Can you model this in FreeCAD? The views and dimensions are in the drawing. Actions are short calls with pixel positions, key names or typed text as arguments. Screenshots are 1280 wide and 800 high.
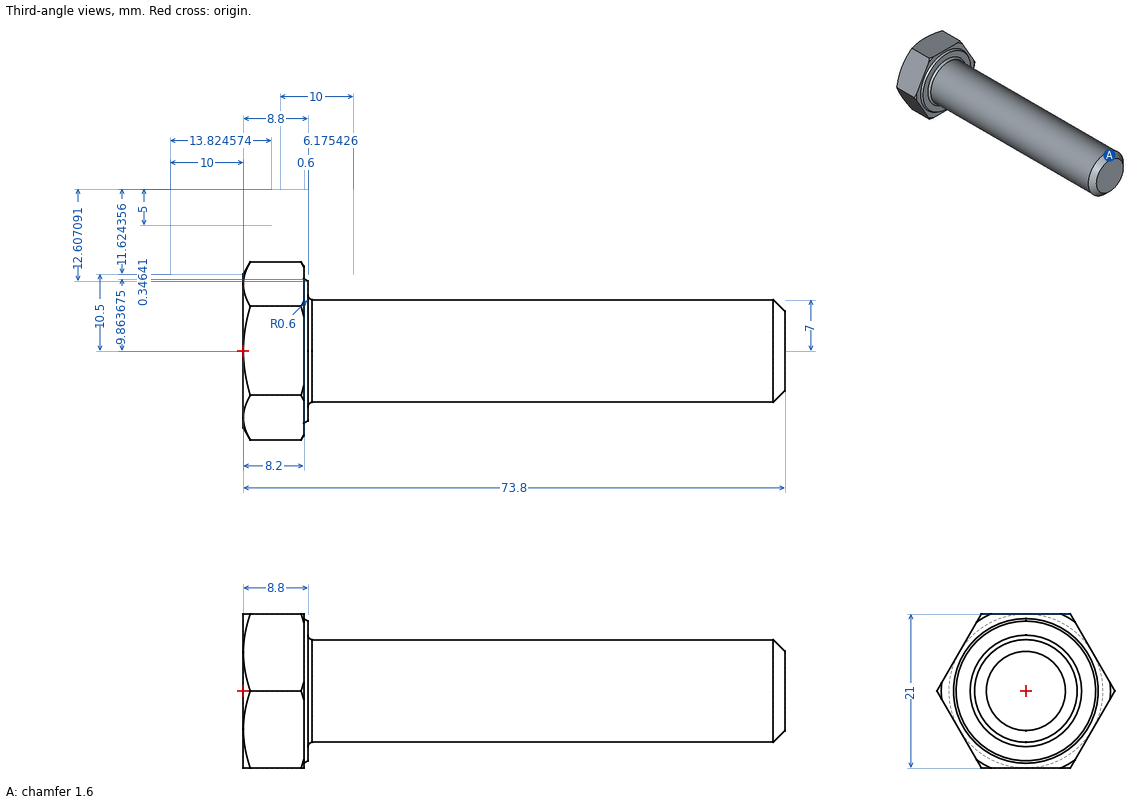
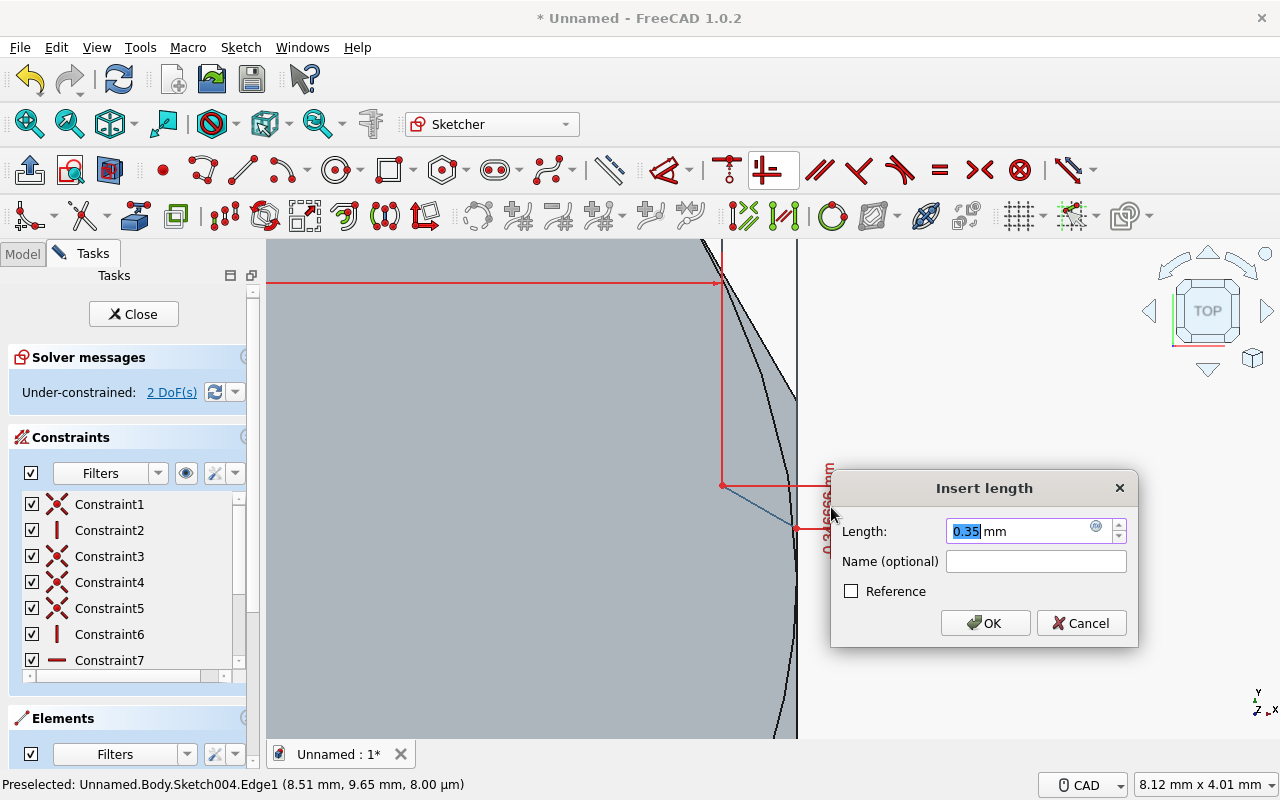
text(0.34641)
key(Return)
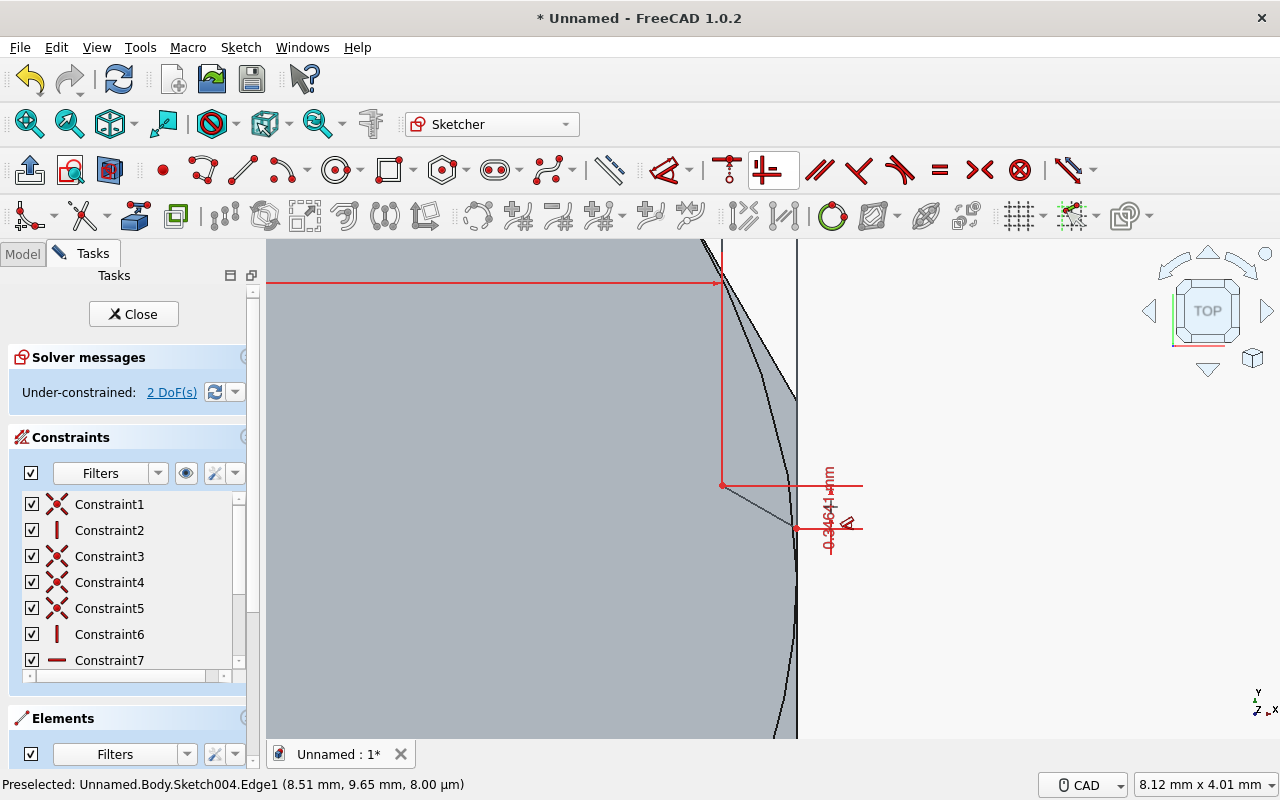
scroll(761, 509, down, 11)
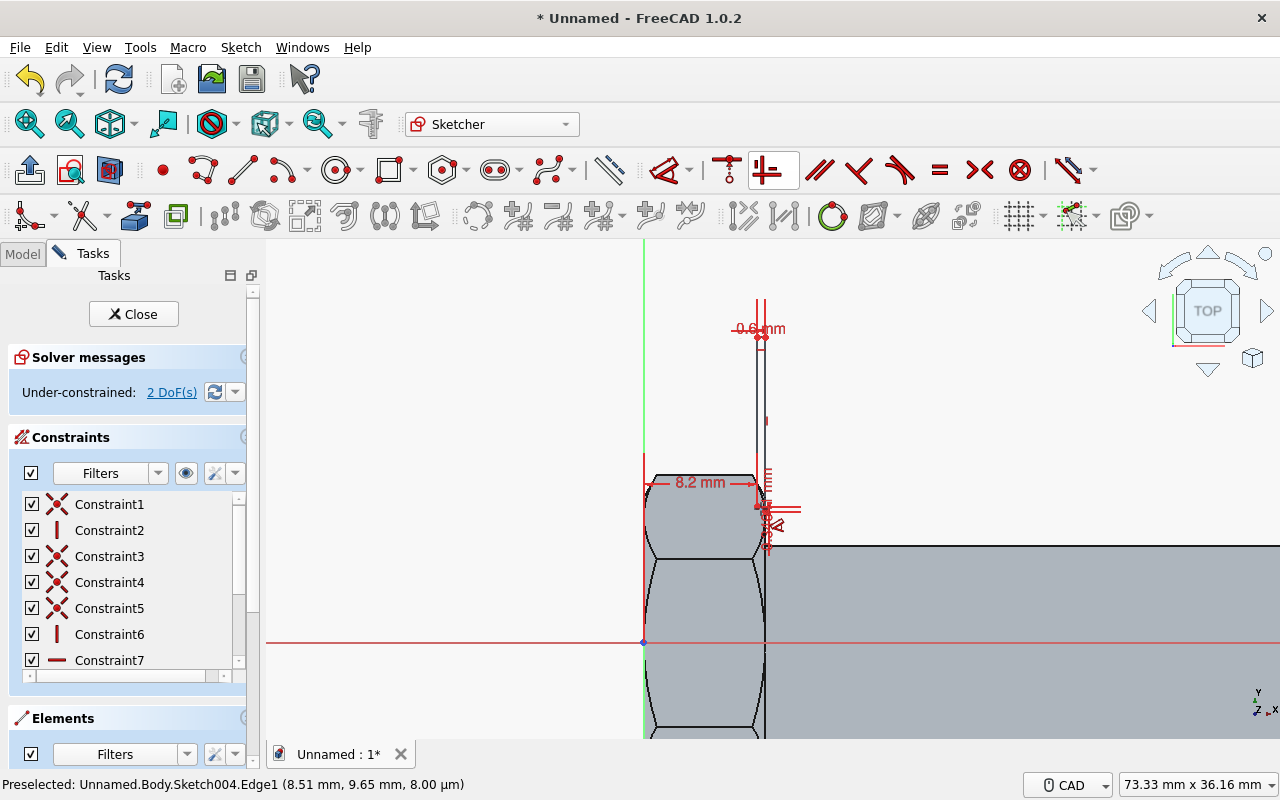
scroll(765, 459, up, 3)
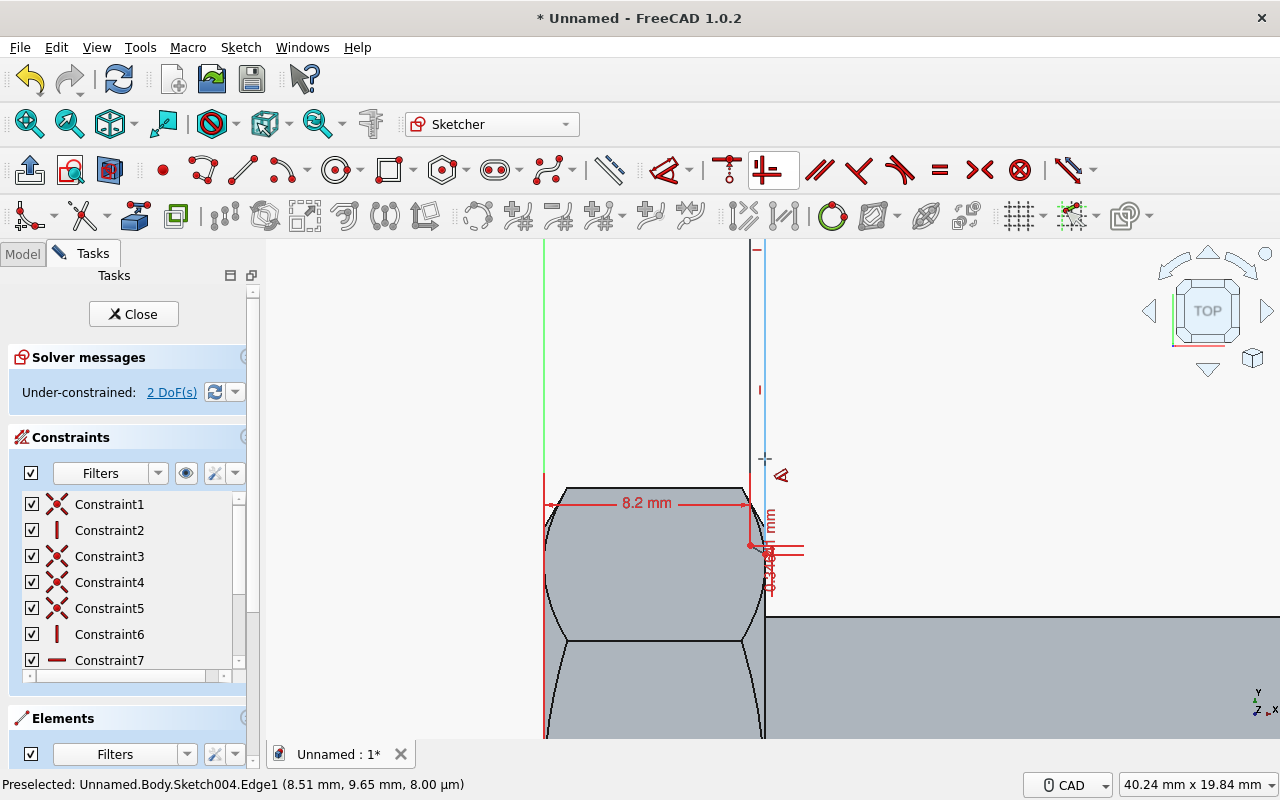
click(765, 459)
click(799, 411)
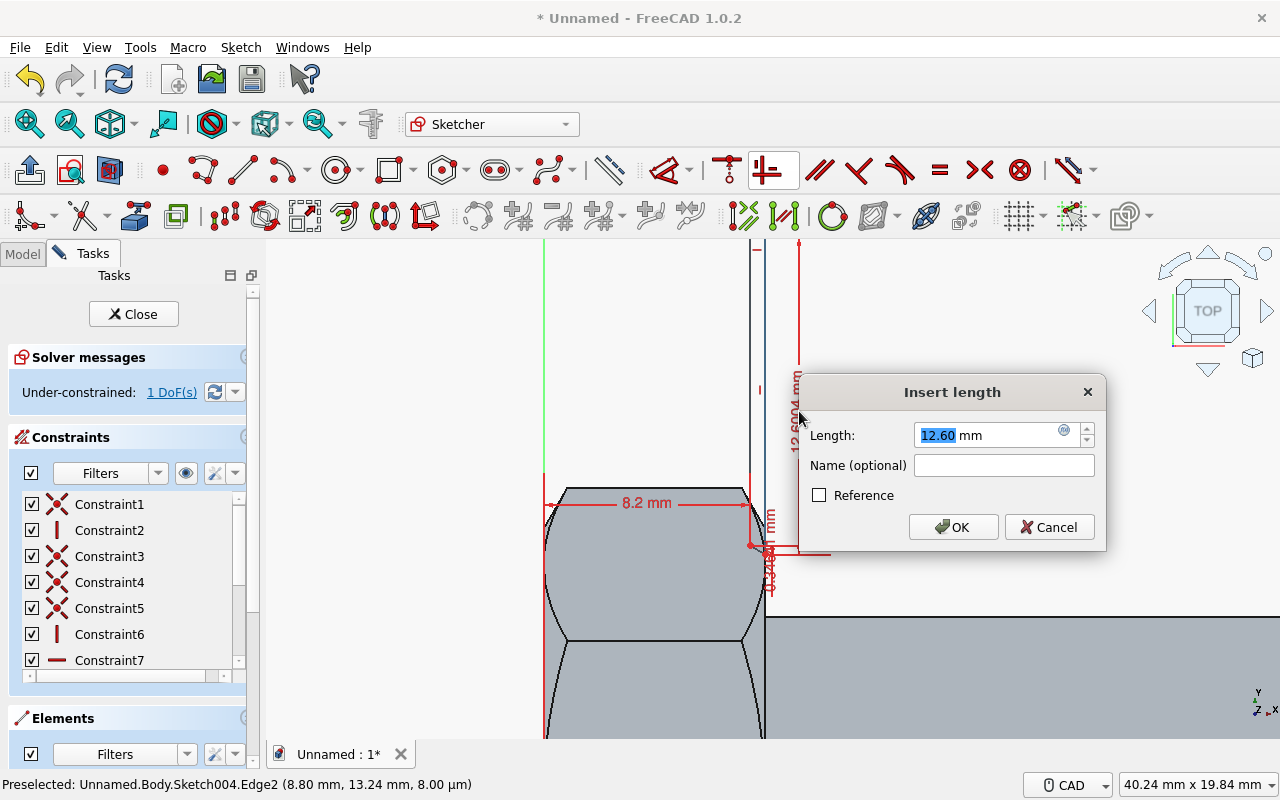
text(12.607091)
key(Return)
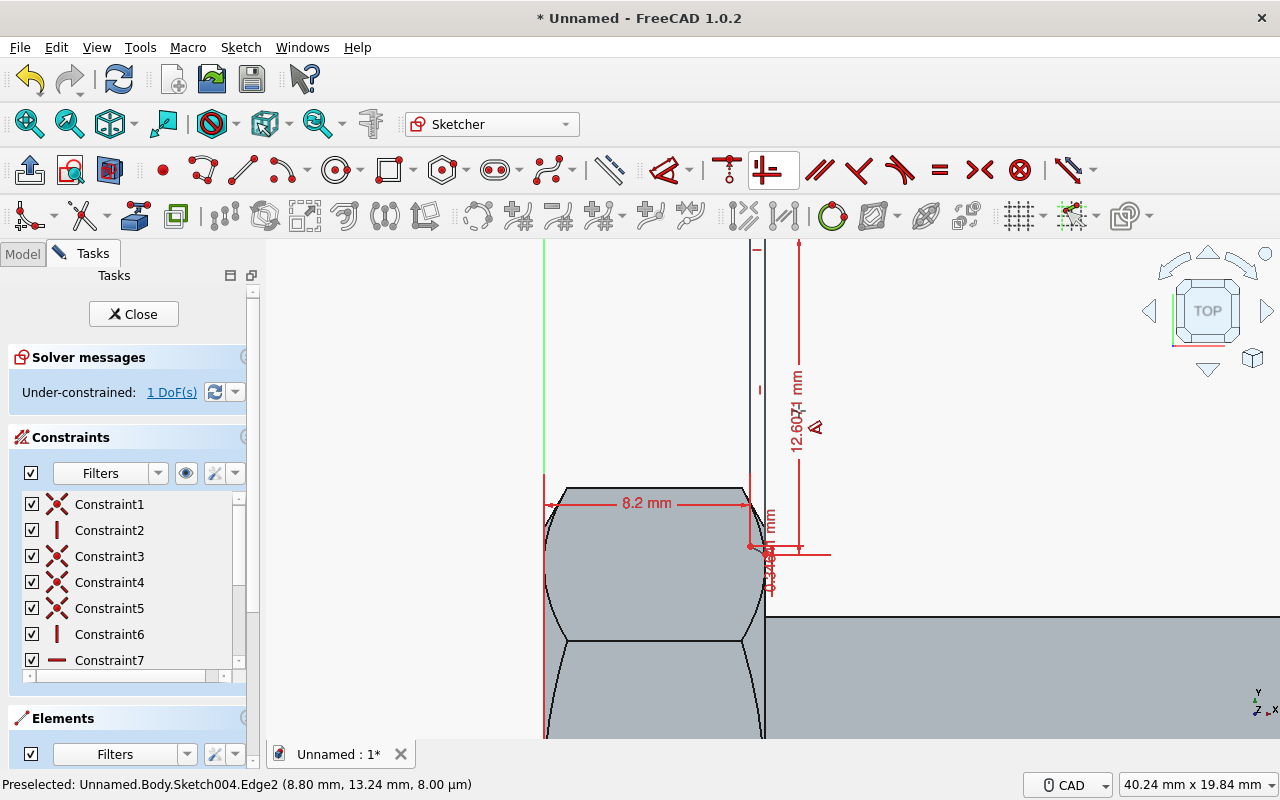
click(750, 546)
click(510, 629)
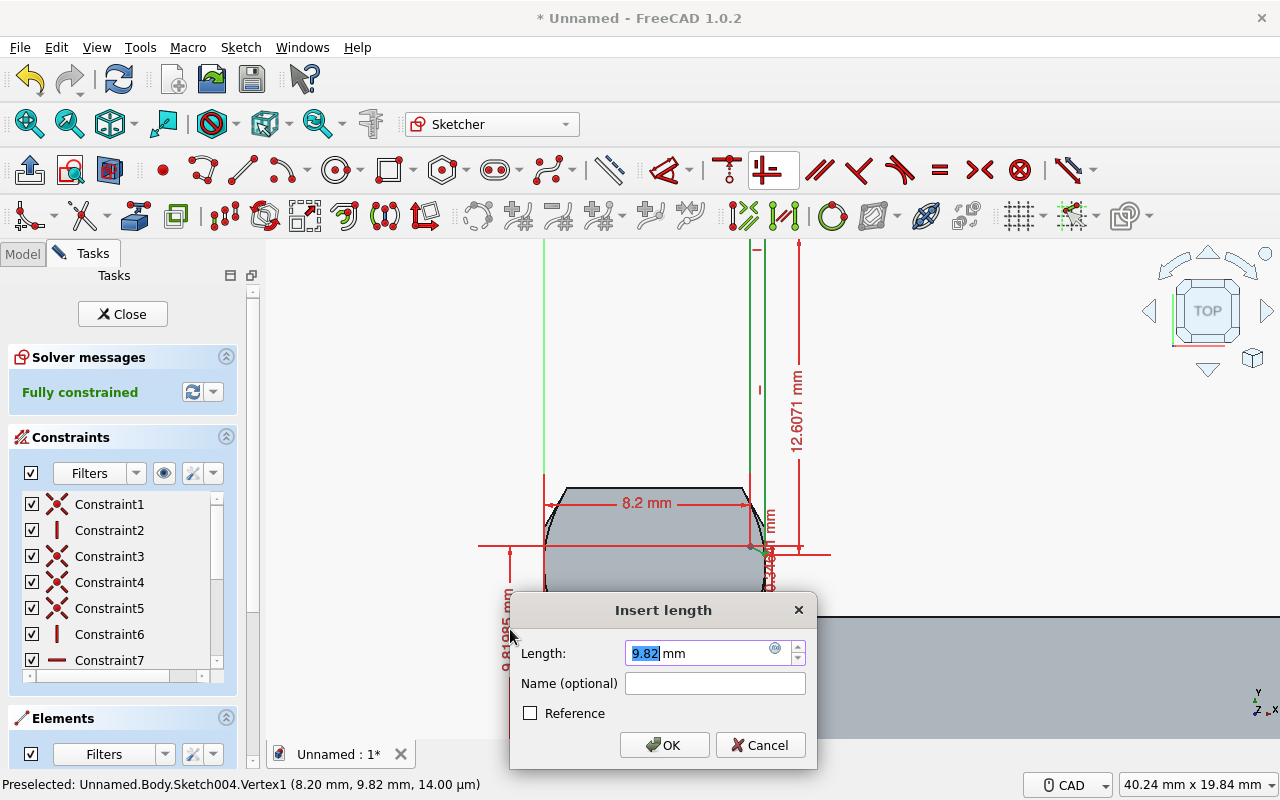
text(9.863675)
key(Return)
key(Escape)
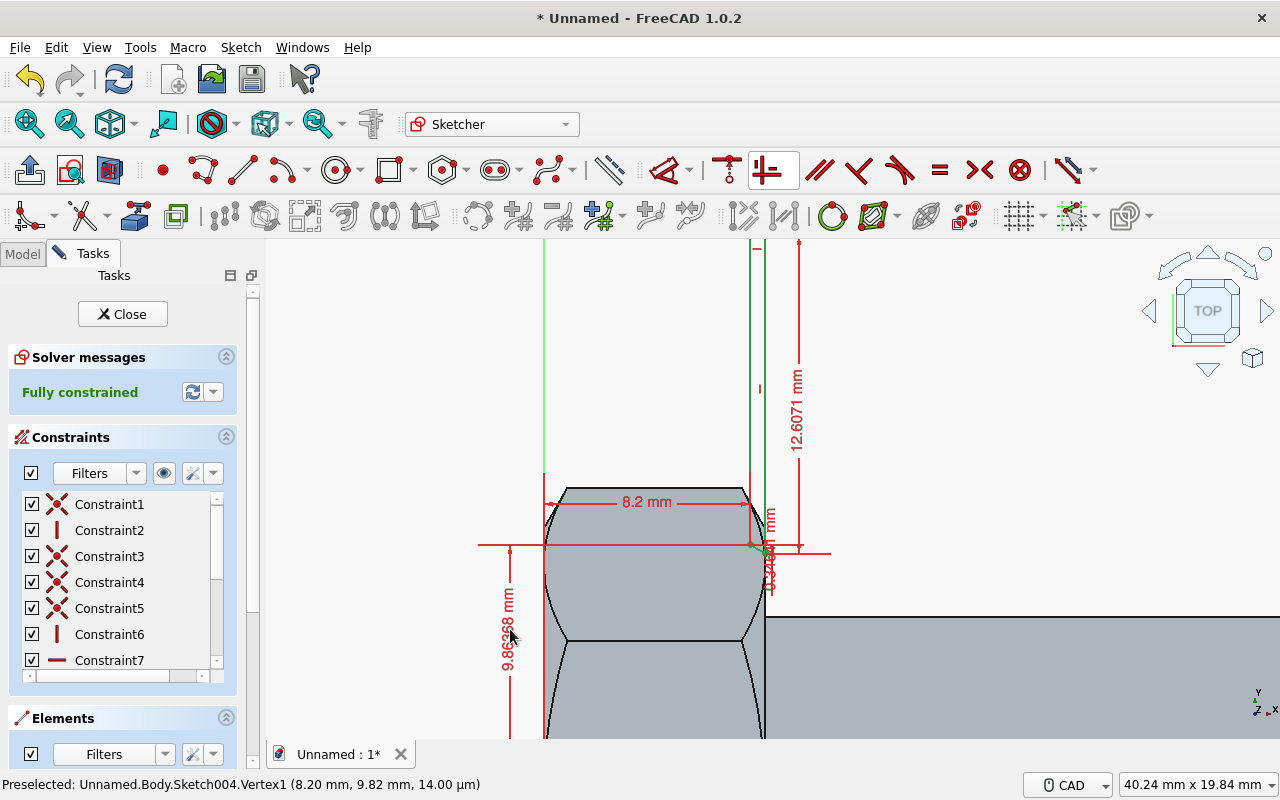
click(123, 314)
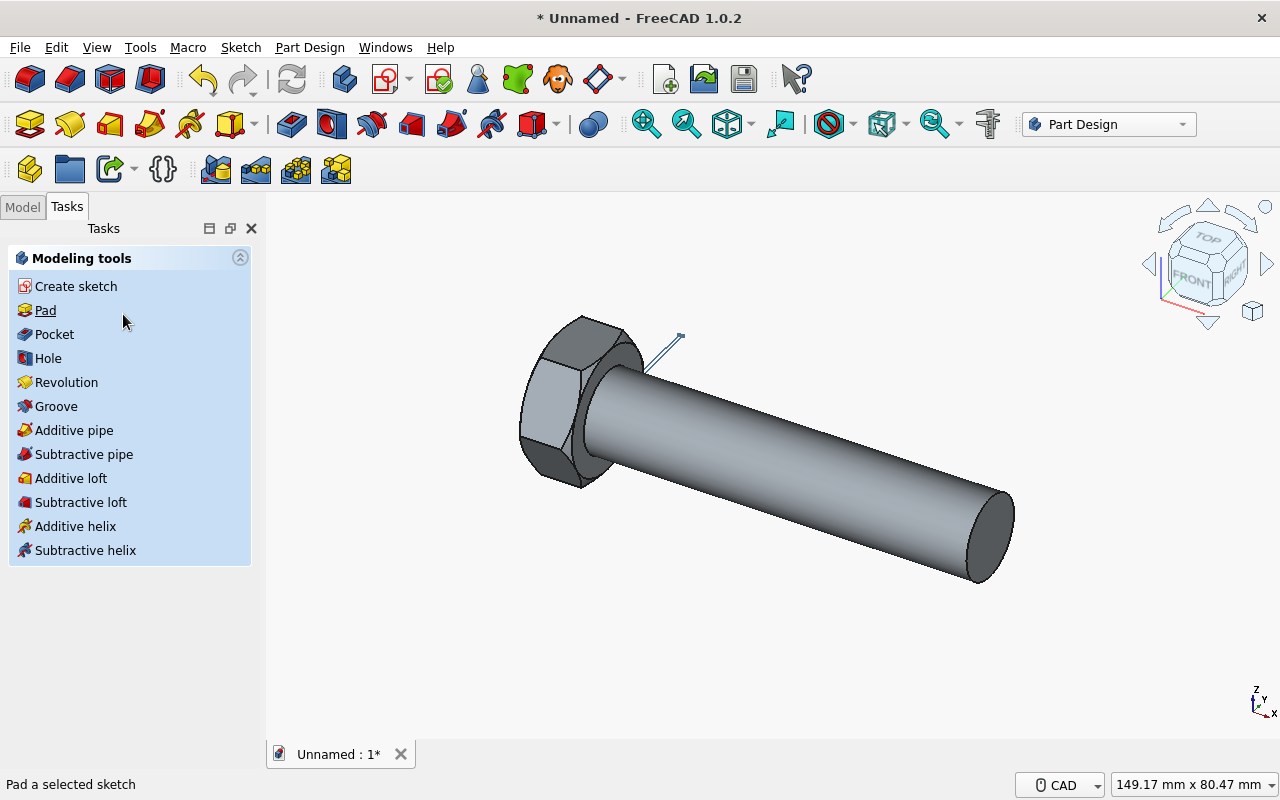
click(372, 124)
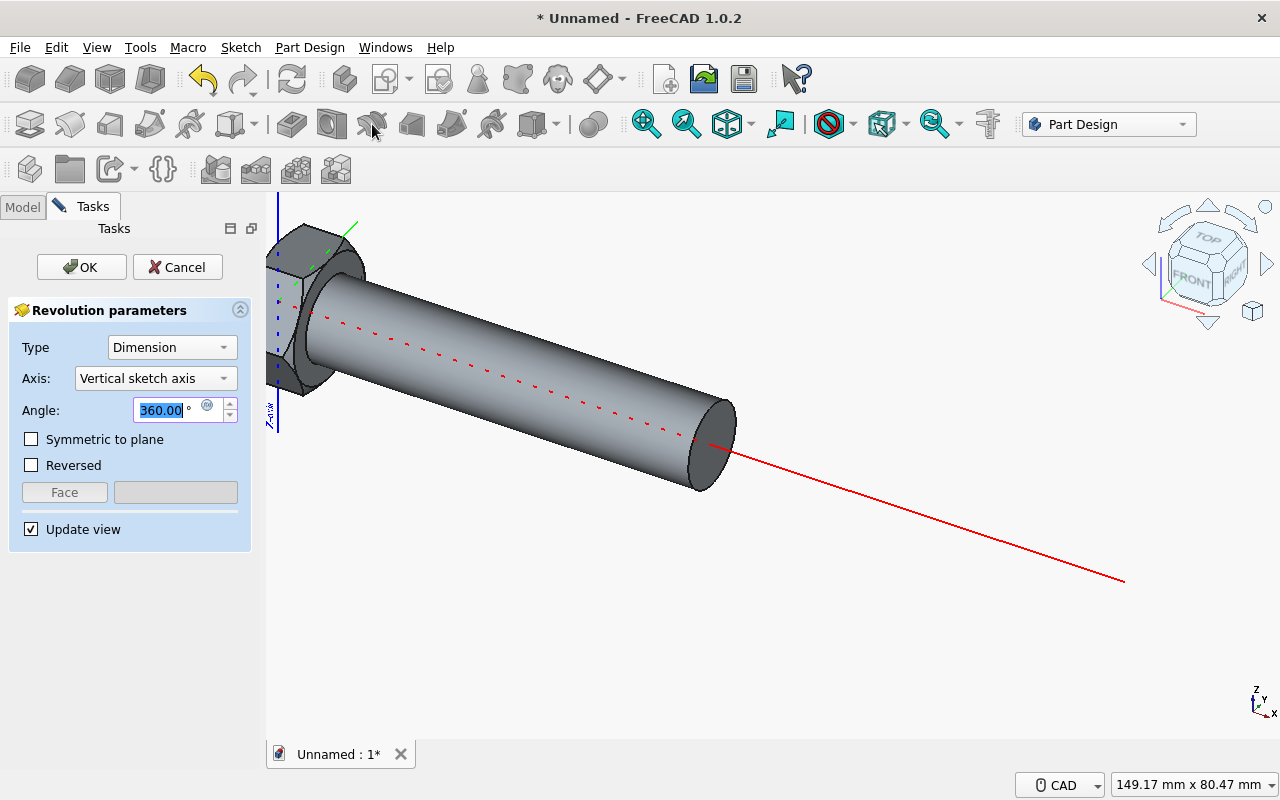
click(156, 378)